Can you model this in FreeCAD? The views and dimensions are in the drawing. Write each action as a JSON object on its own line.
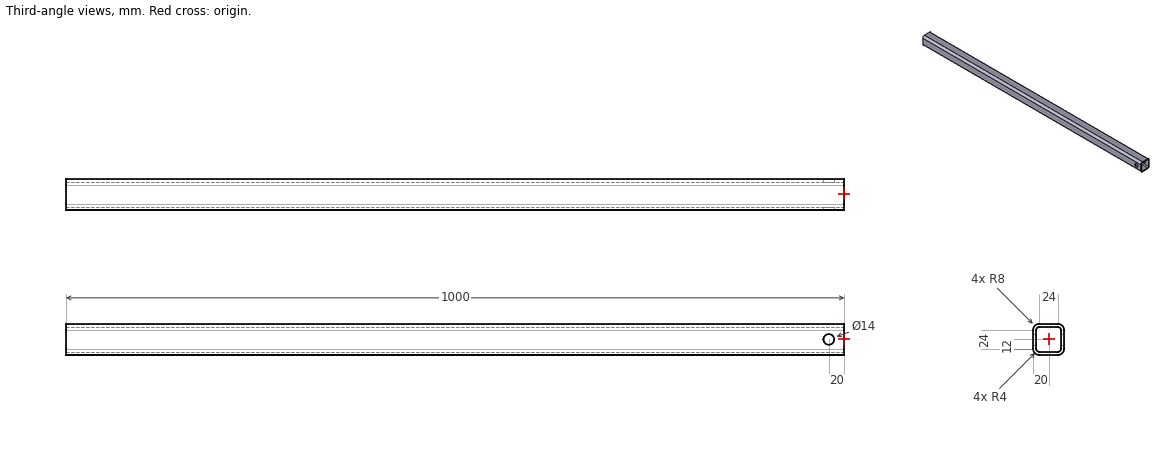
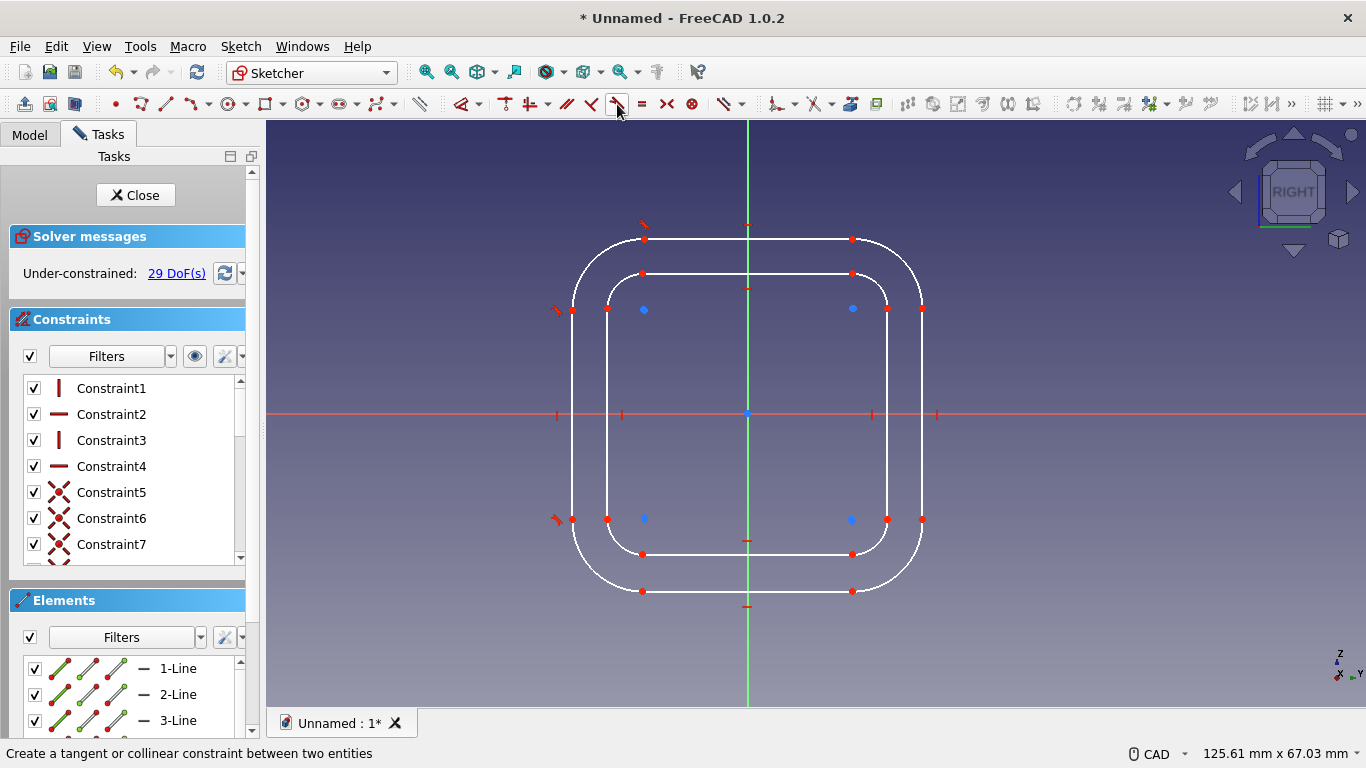
{"action": "left_click", "coordinate": [707, 239]}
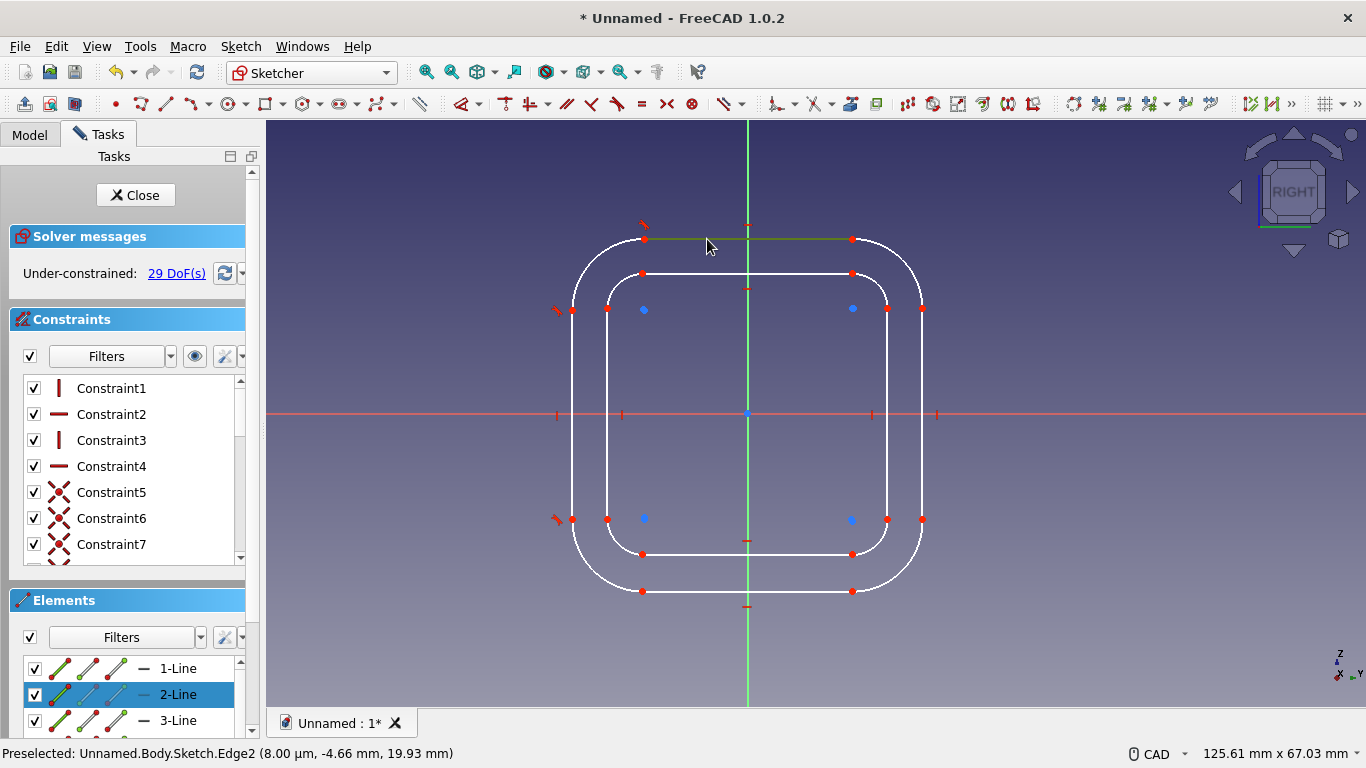
{"action": "left_click", "coordinate": [915, 277]}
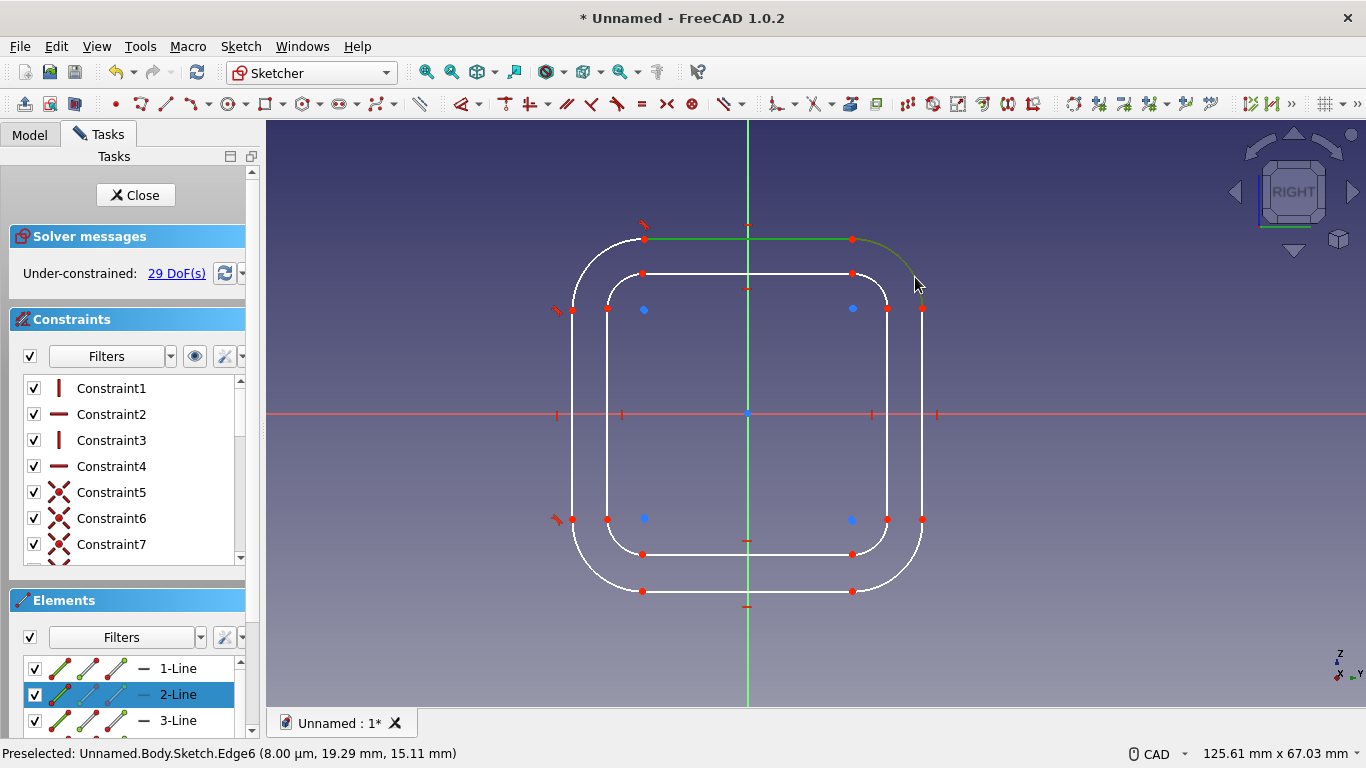
{"action": "left_click", "coordinate": [617, 104]}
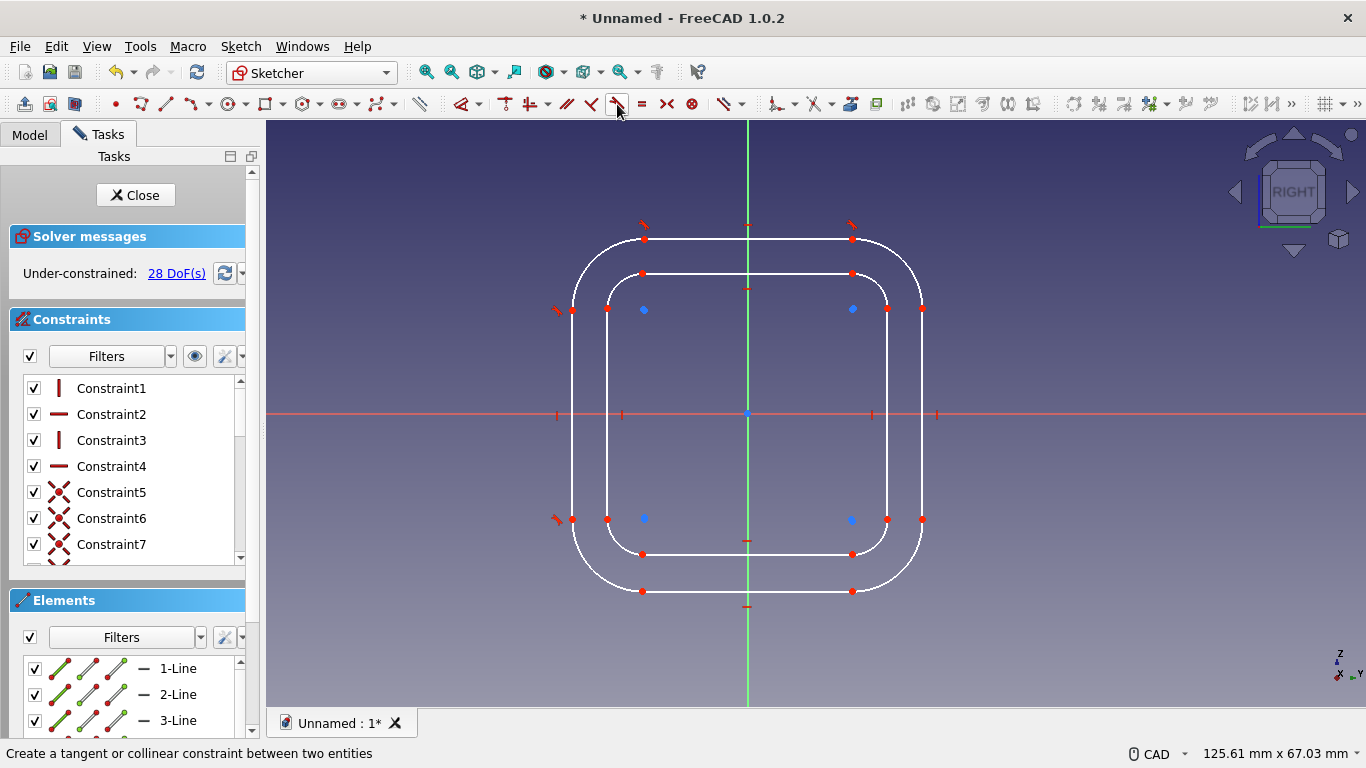
{"action": "left_click", "coordinate": [922, 372]}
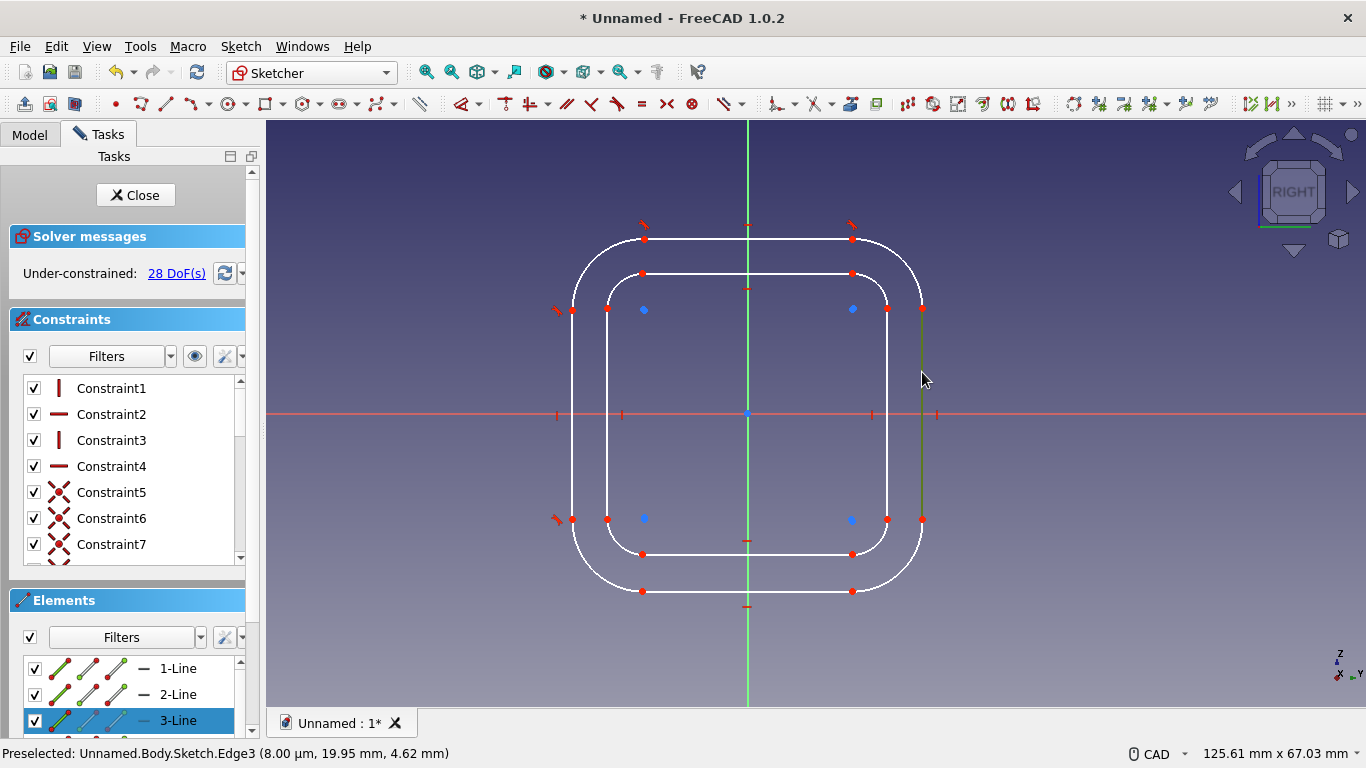
{"action": "left_click", "coordinate": [915, 277]}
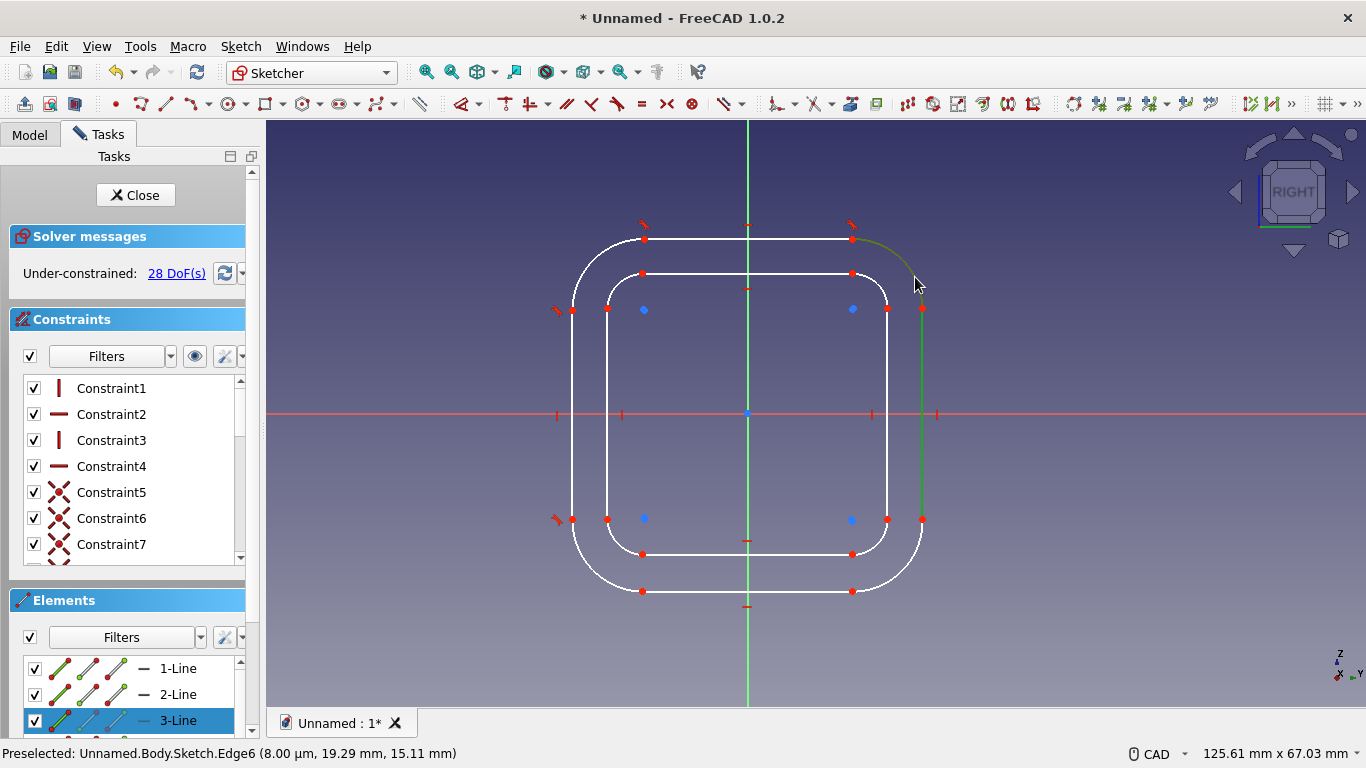
{"action": "key", "text": "t"}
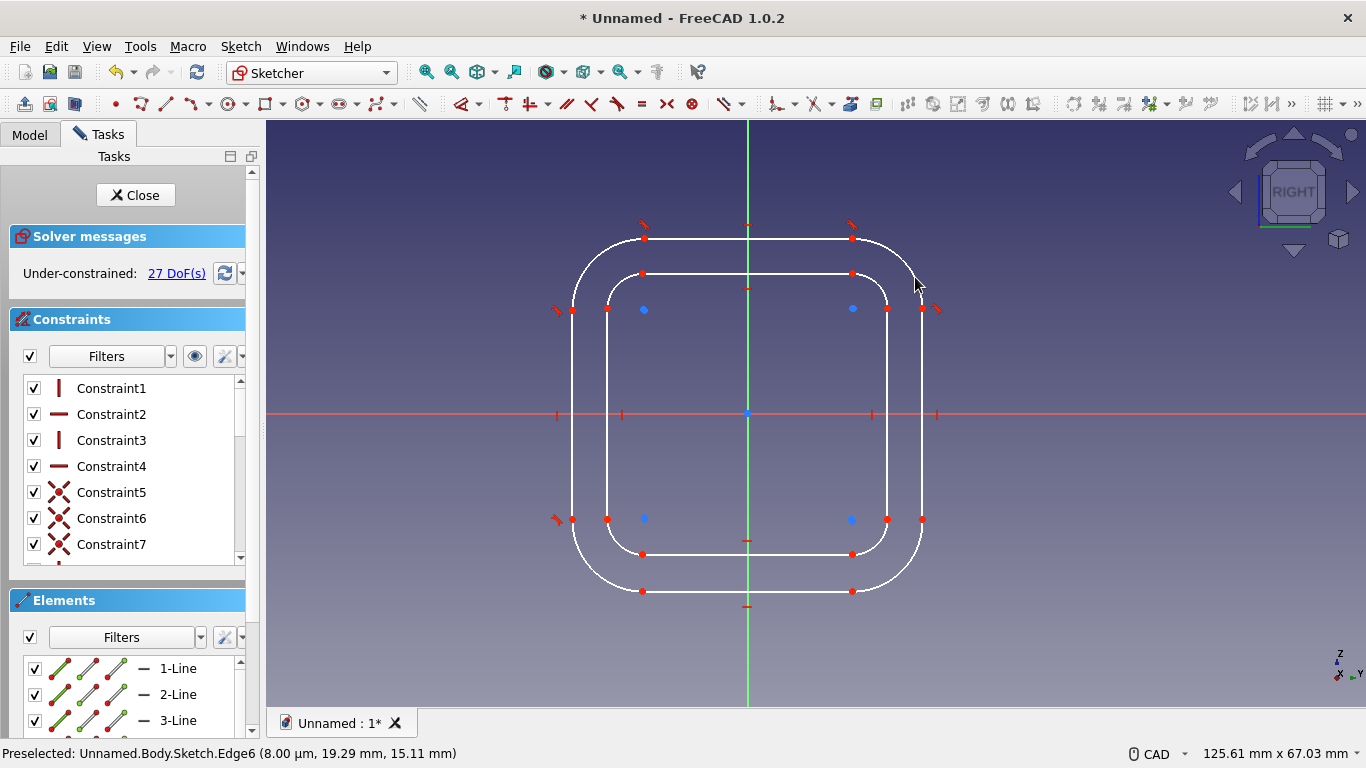
{"action": "left_click", "coordinate": [922, 372]}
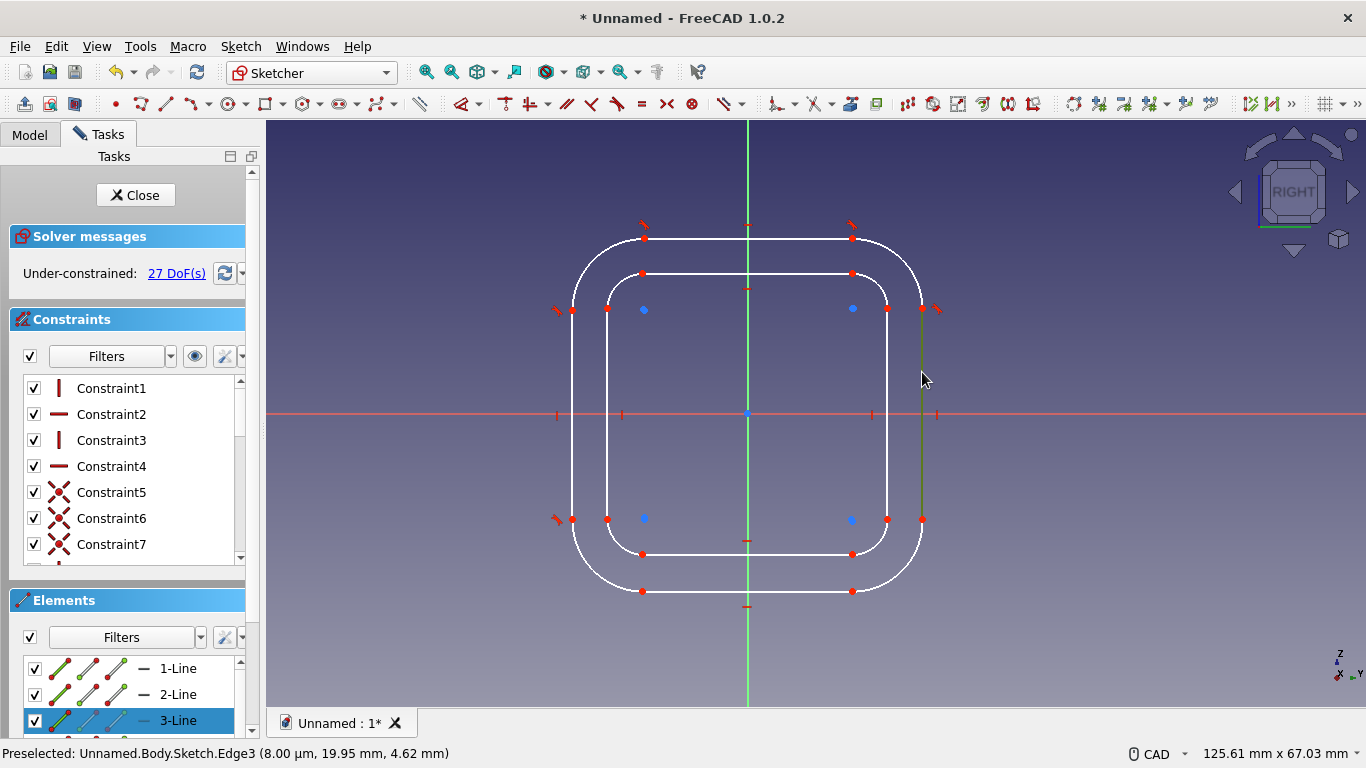
{"action": "left_click", "coordinate": [885, 584]}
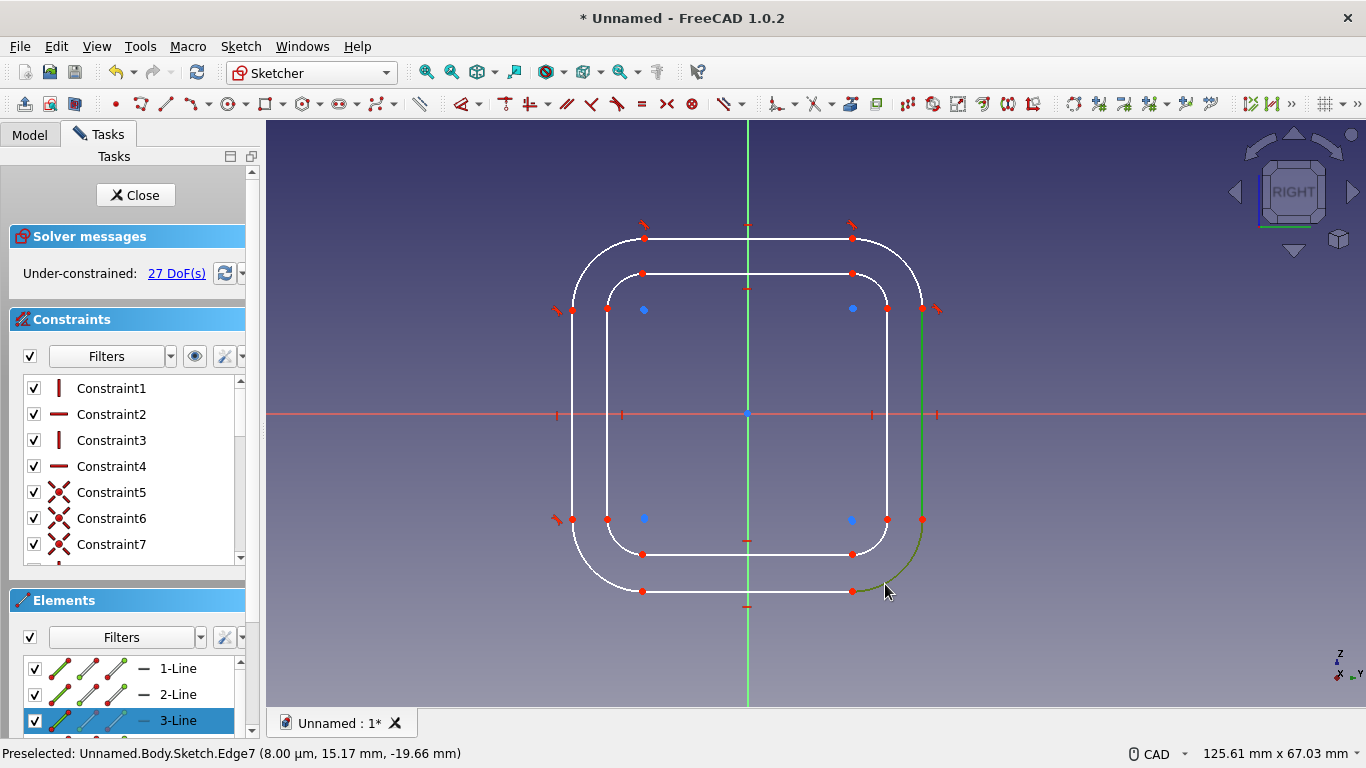
{"action": "left_click", "coordinate": [617, 104]}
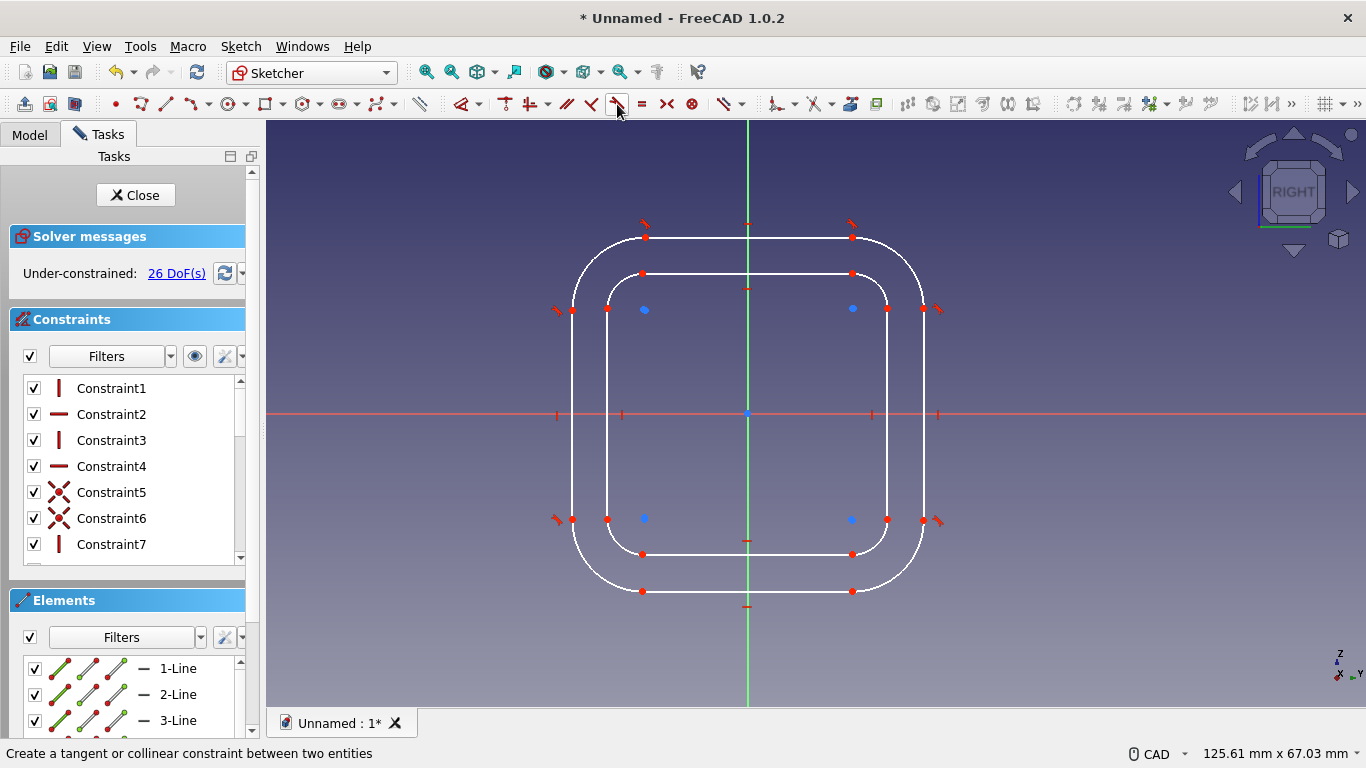
{"action": "left_click", "coordinate": [789, 592]}